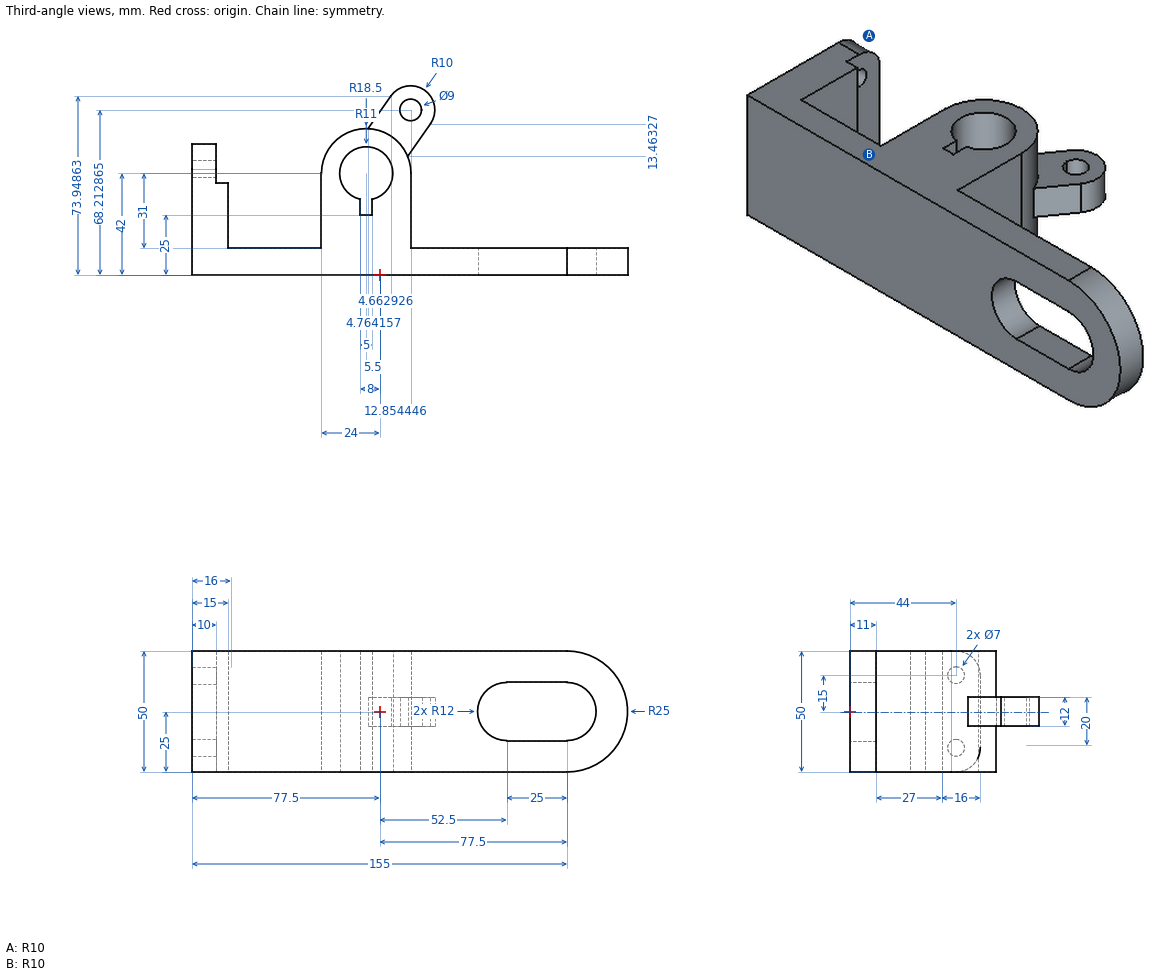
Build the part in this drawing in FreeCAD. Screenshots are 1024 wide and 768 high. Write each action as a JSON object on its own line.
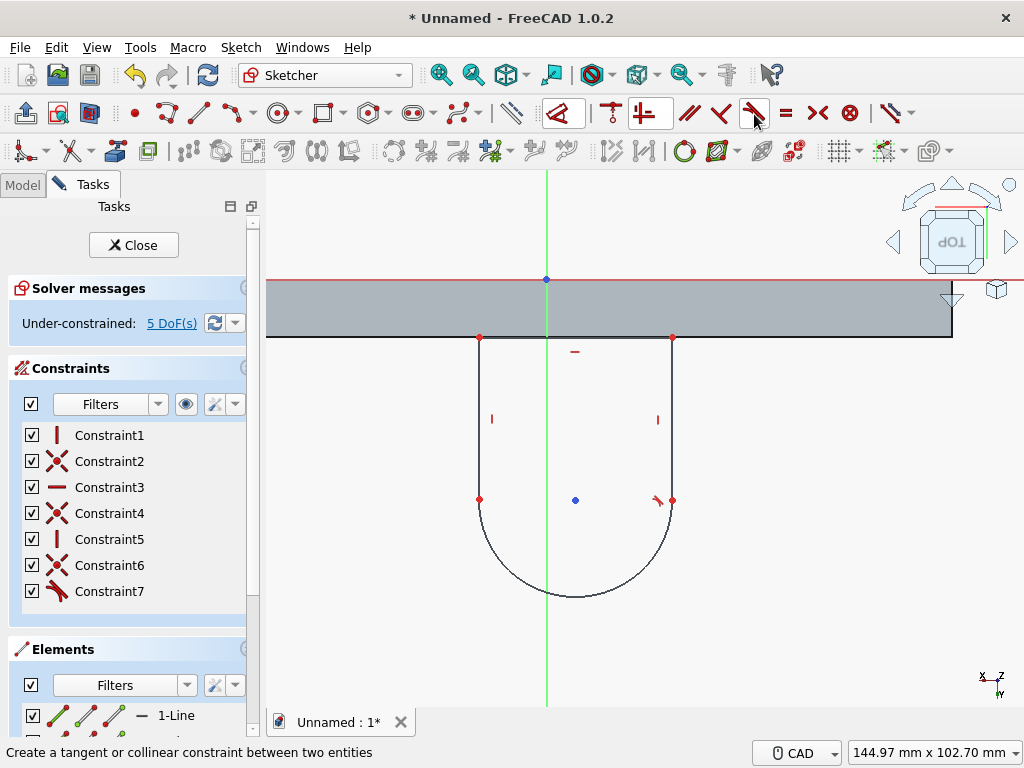
{"action": "left_click", "coordinate": [479, 387]}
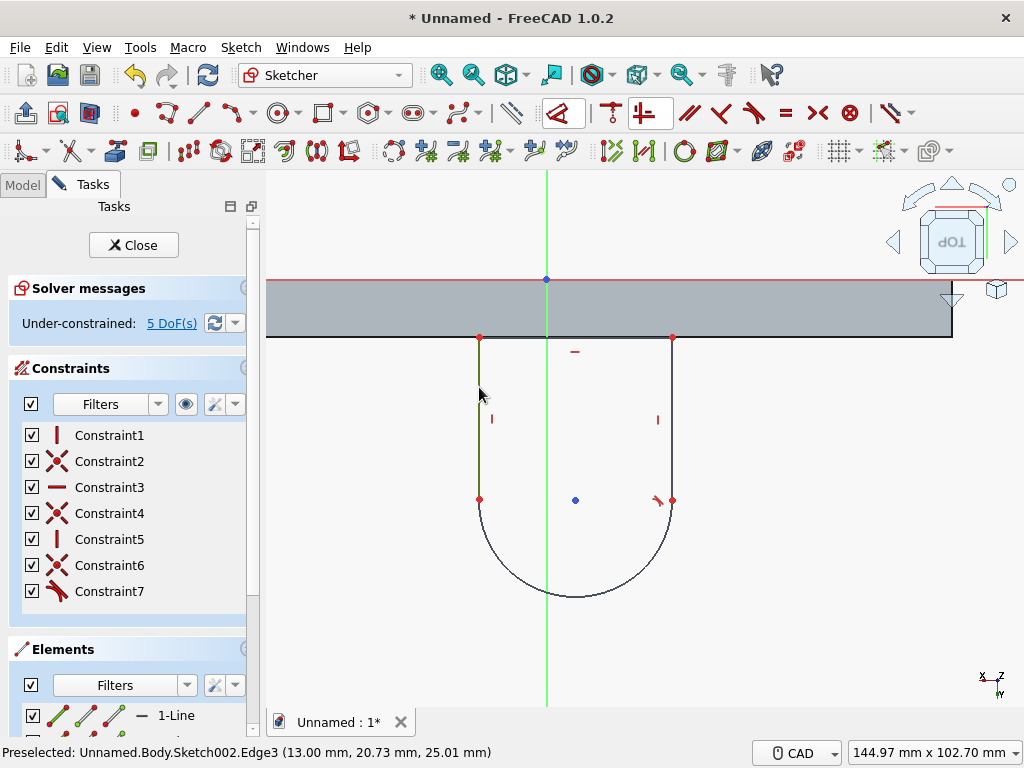
{"action": "left_click", "coordinate": [518, 578]}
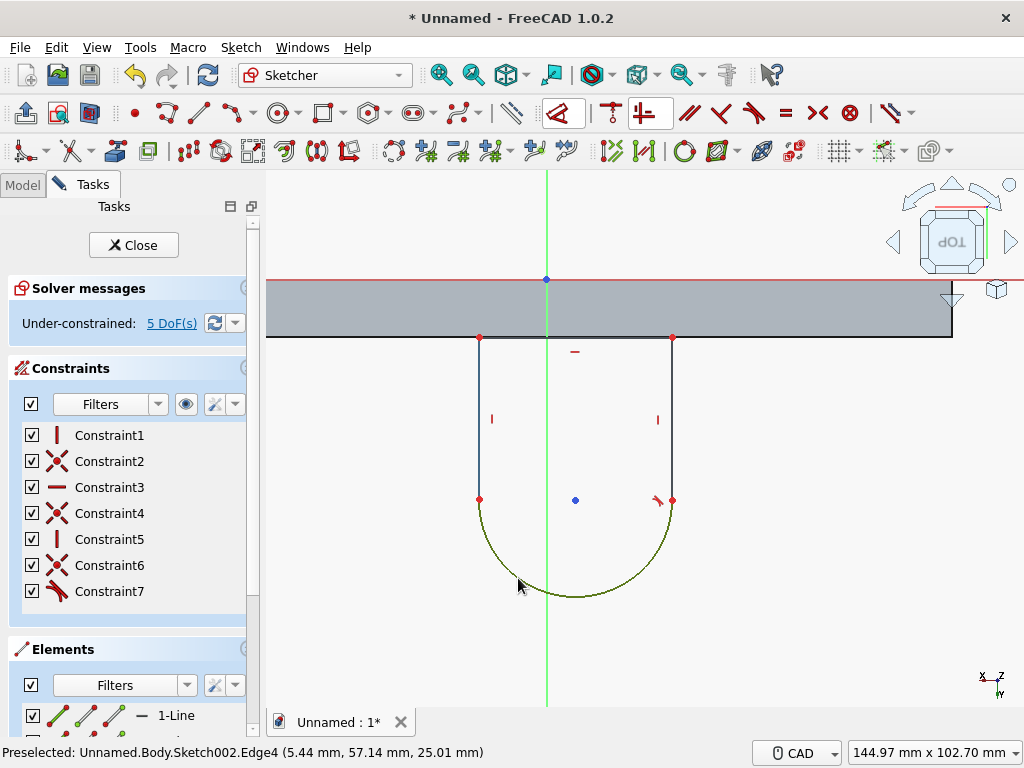
{"action": "left_click", "coordinate": [754, 114]}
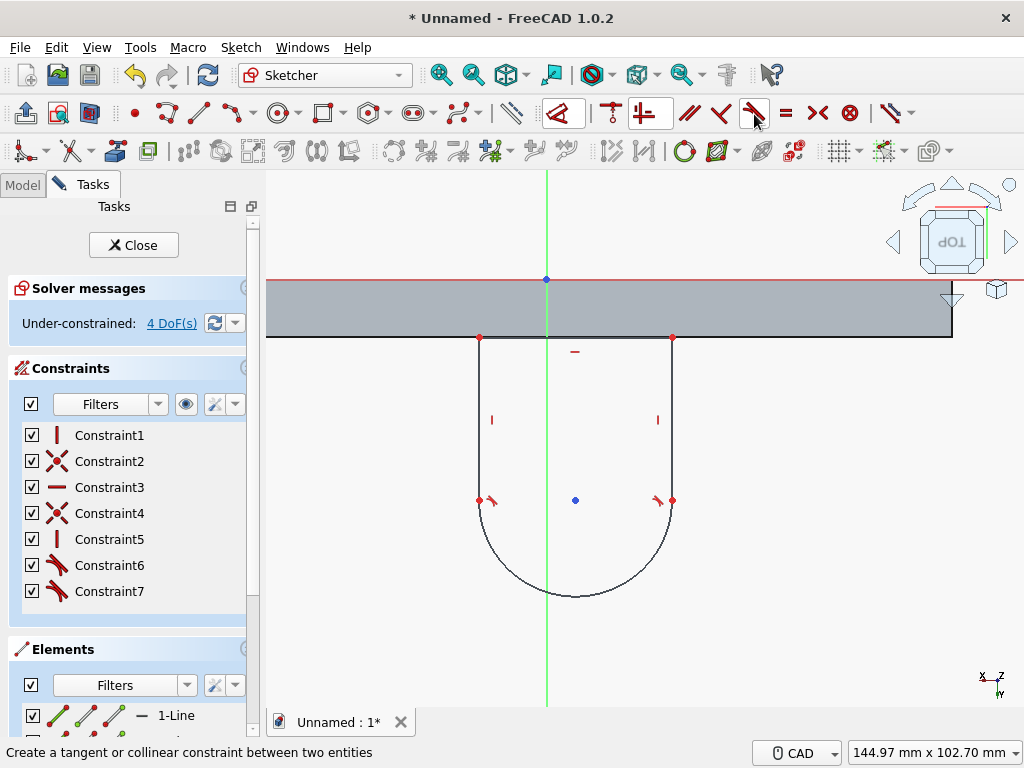
{"action": "left_click", "coordinate": [519, 578]}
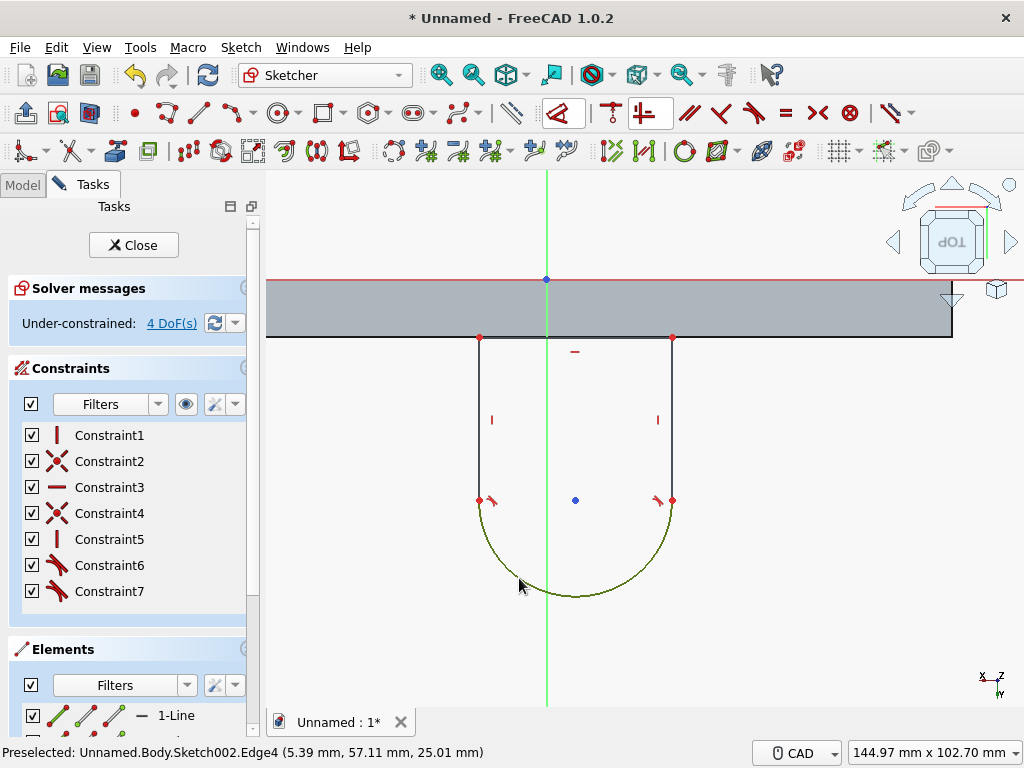
{"action": "left_click", "coordinate": [580, 114]}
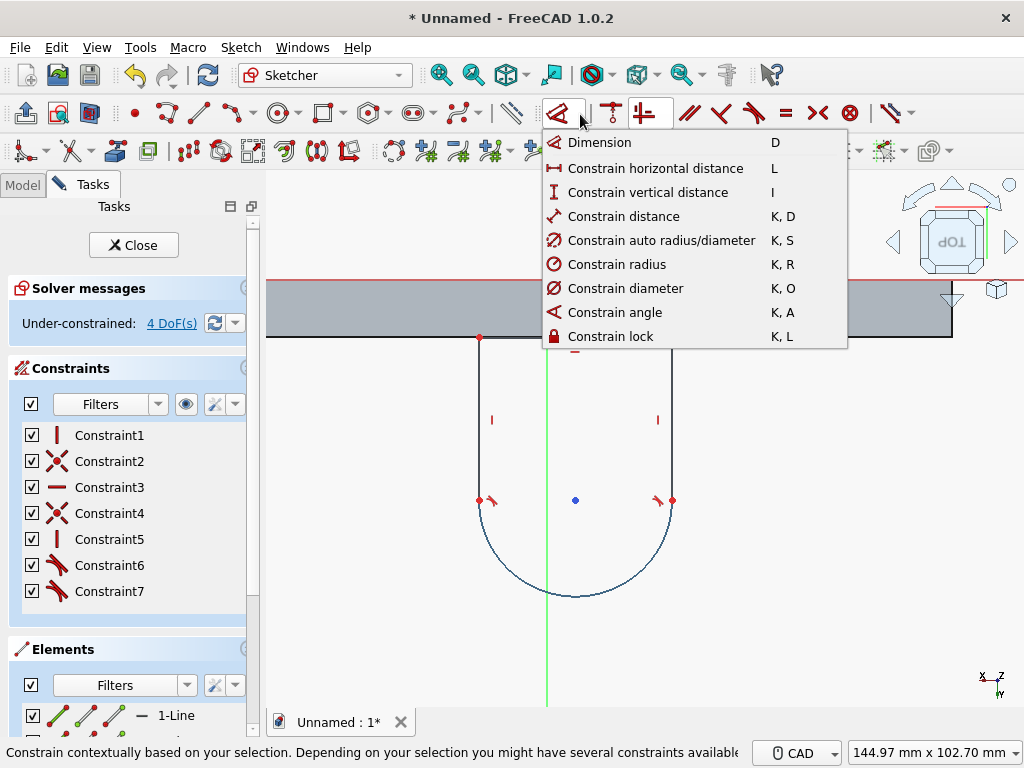
{"action": "left_click", "coordinate": [695, 264]}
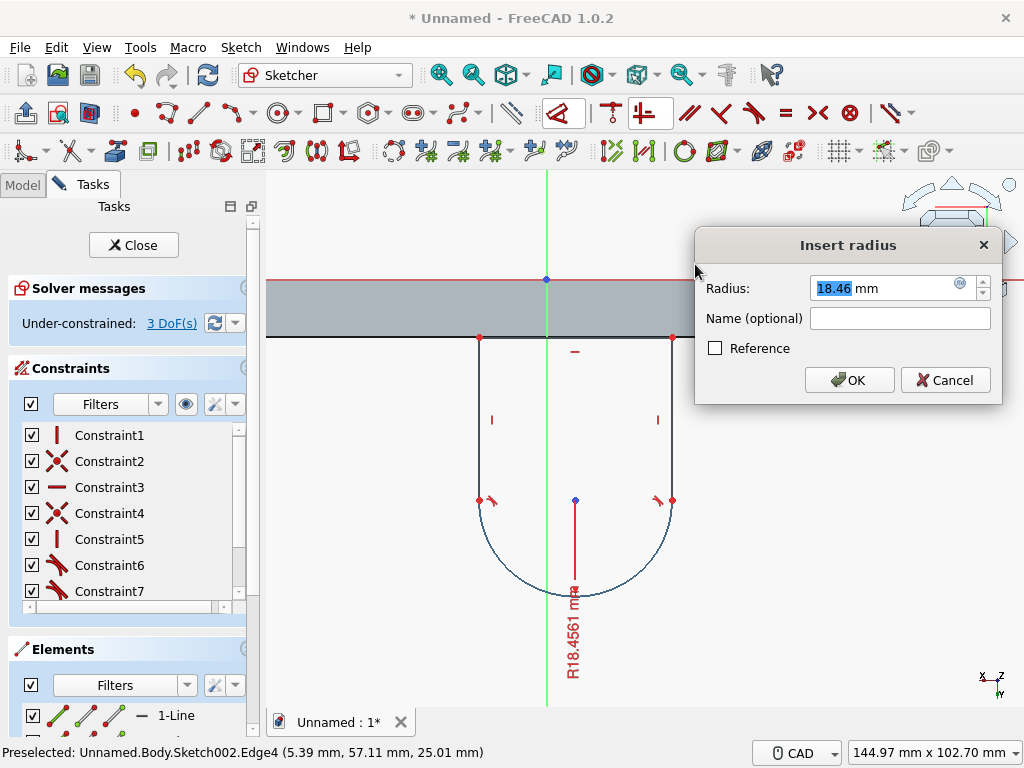
{"action": "type", "text": "18.5"}
{"action": "key", "text": "Return"}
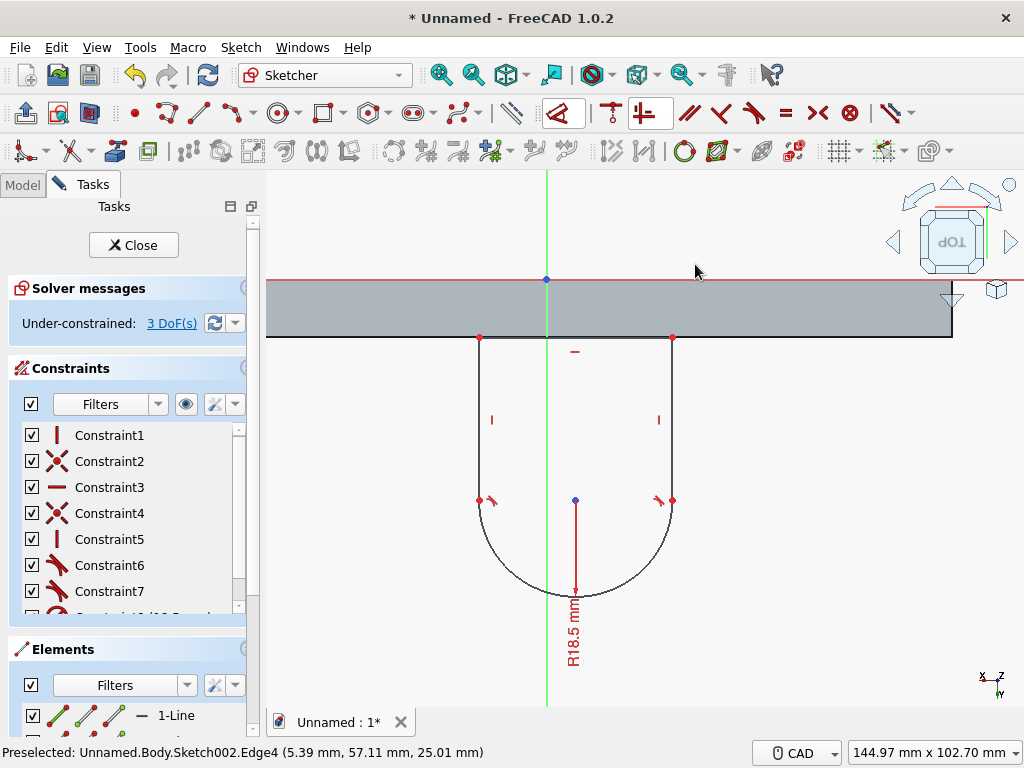
{"action": "left_click", "coordinate": [672, 451]}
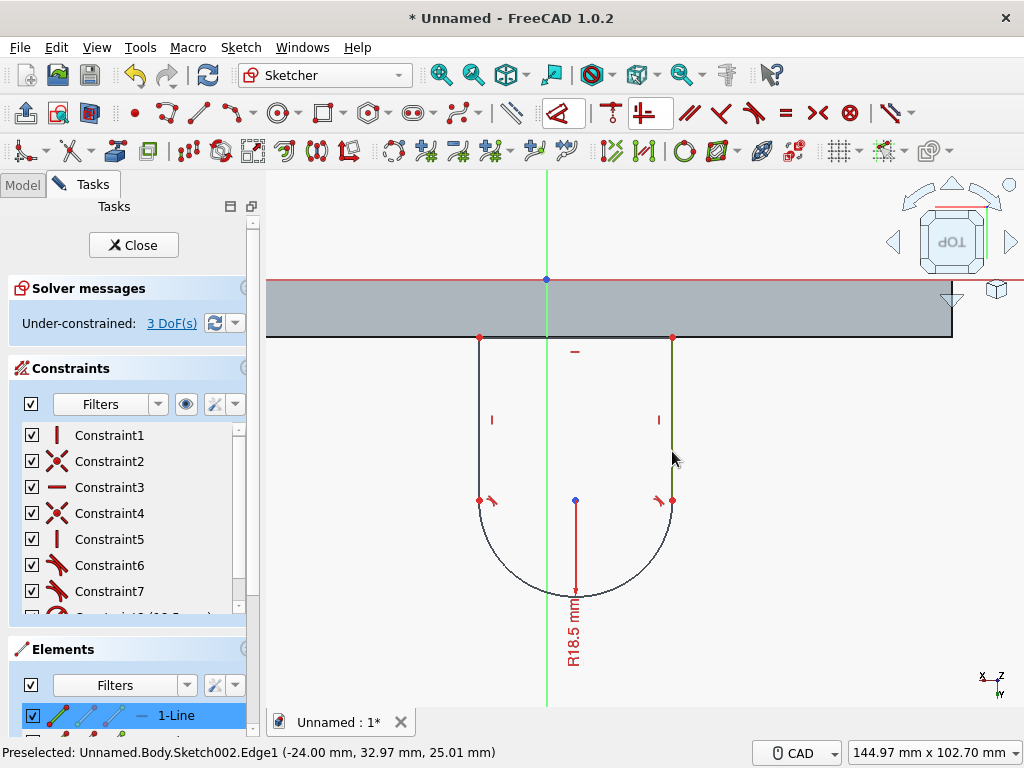
{"action": "key", "text": "i"}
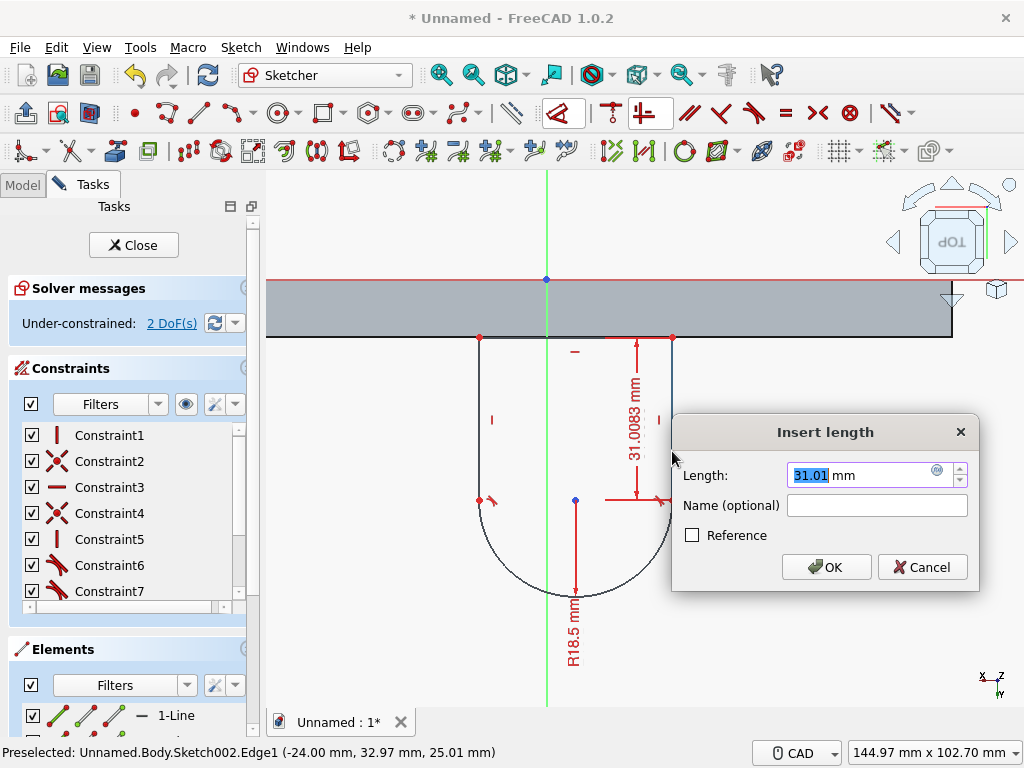
{"action": "type", "text": "31"}
{"action": "key", "text": "Return"}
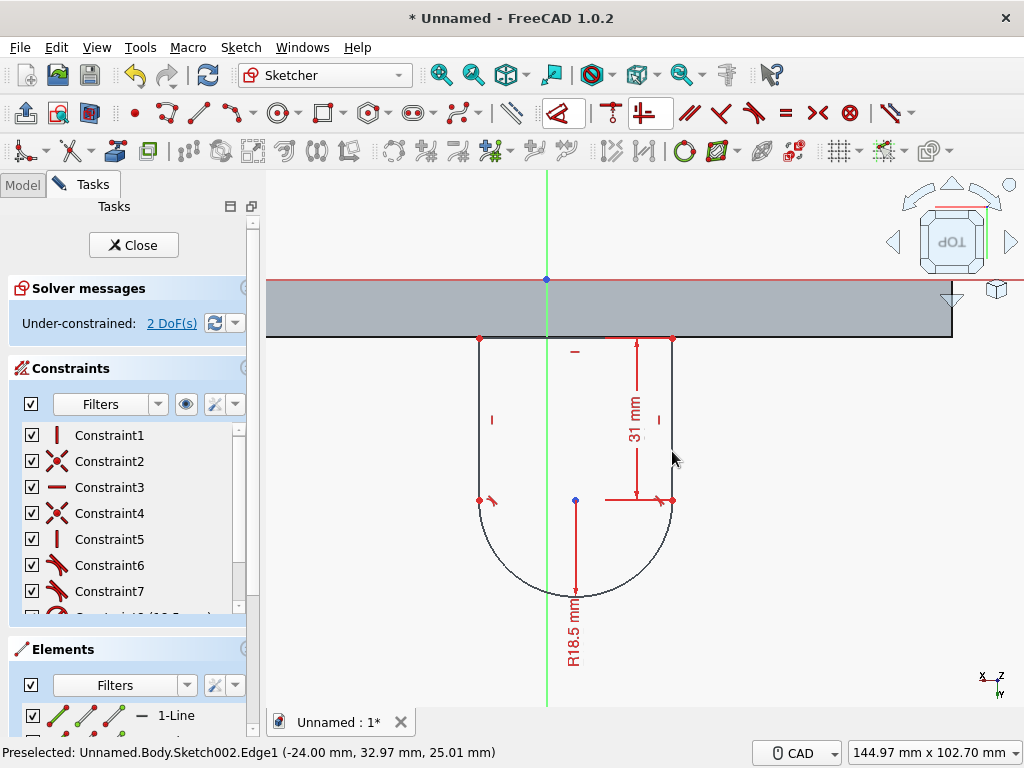
{"action": "left_click", "coordinate": [672, 500]}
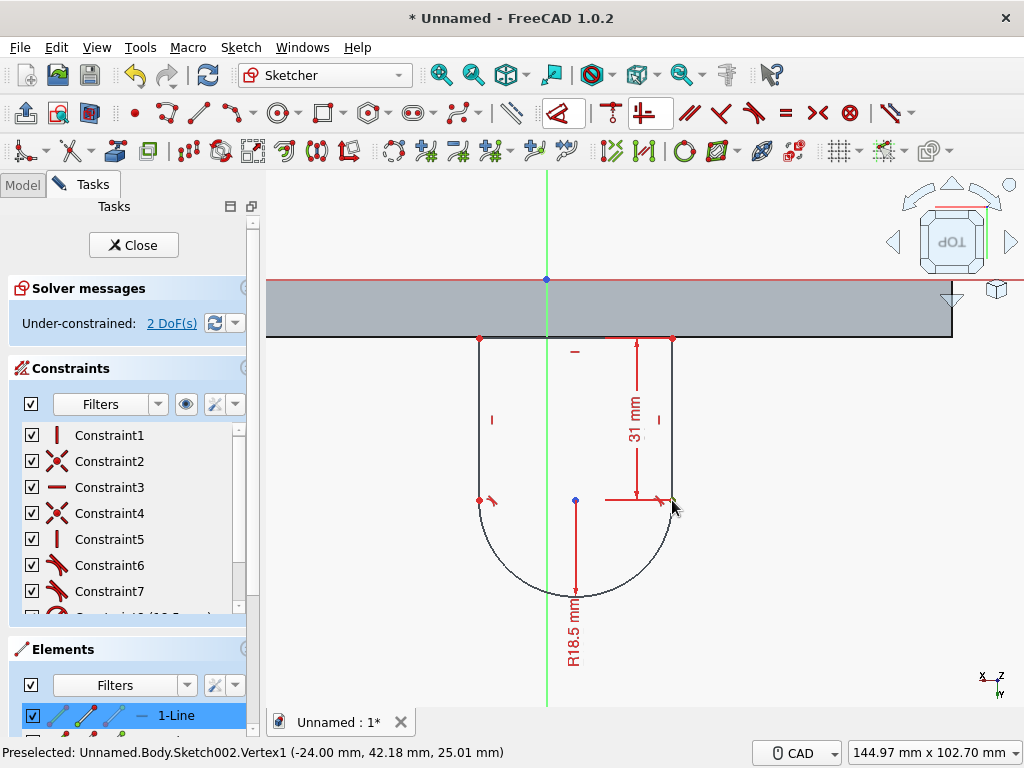
{"action": "key", "text": "l"}